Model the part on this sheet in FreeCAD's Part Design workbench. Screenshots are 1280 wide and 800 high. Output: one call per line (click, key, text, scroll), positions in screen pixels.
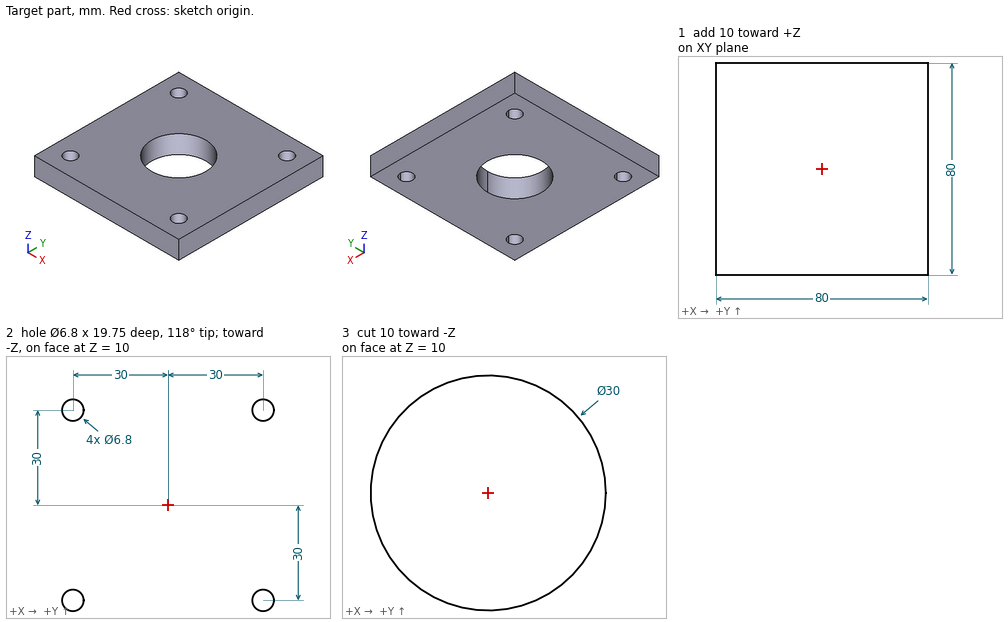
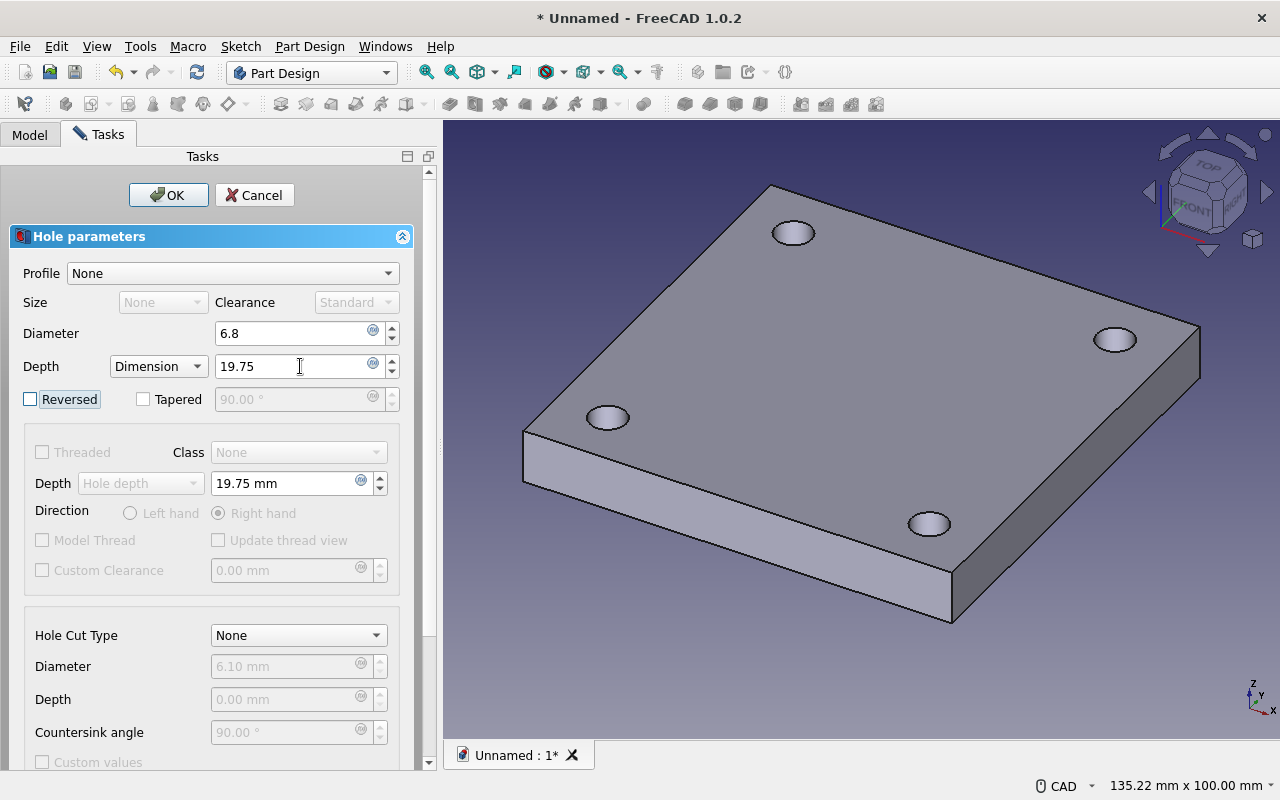
click(169, 195)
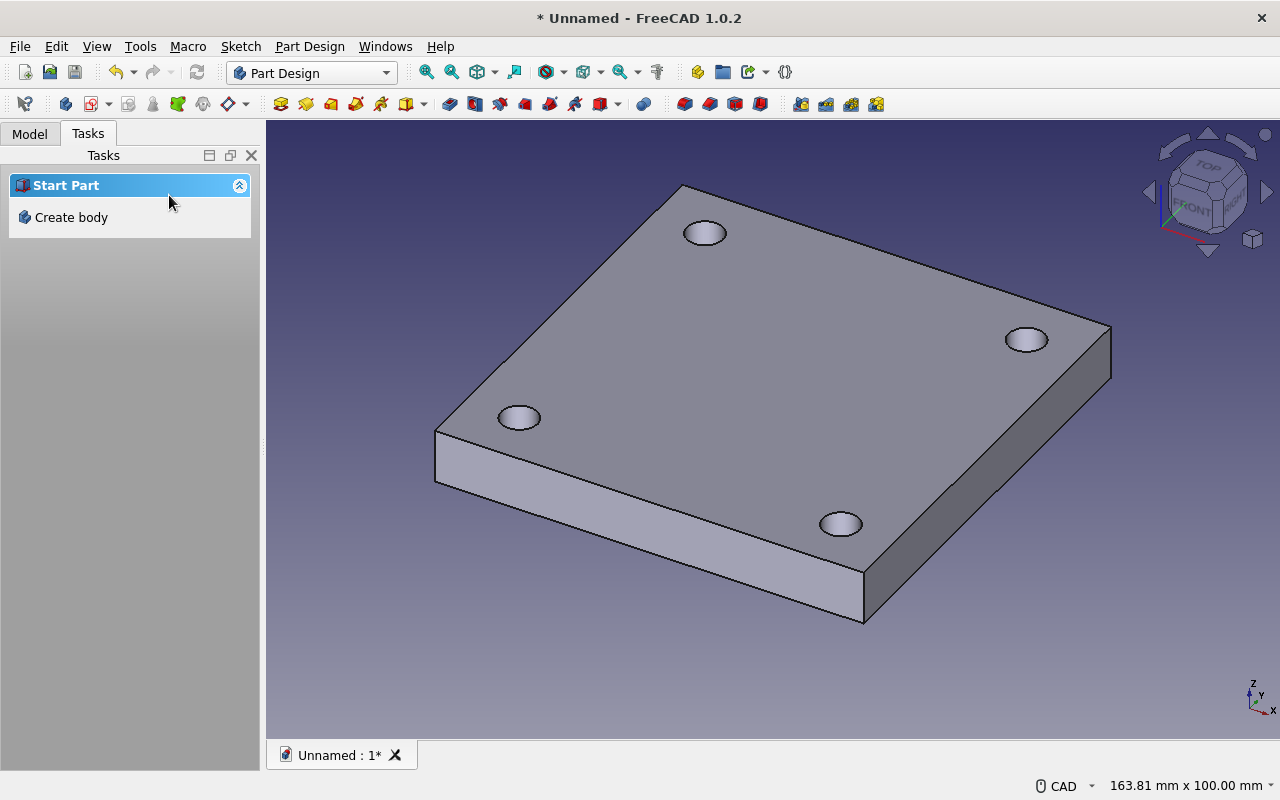
click(773, 378)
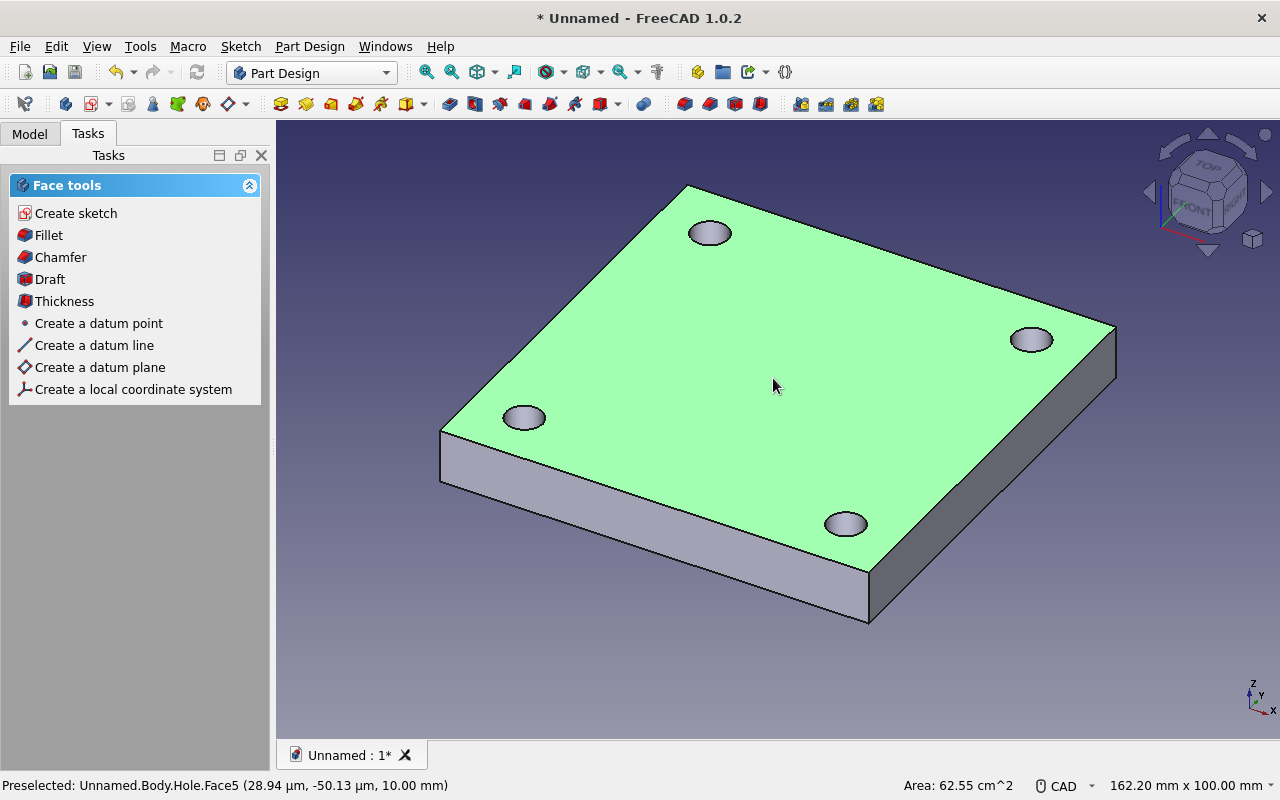
click(90, 104)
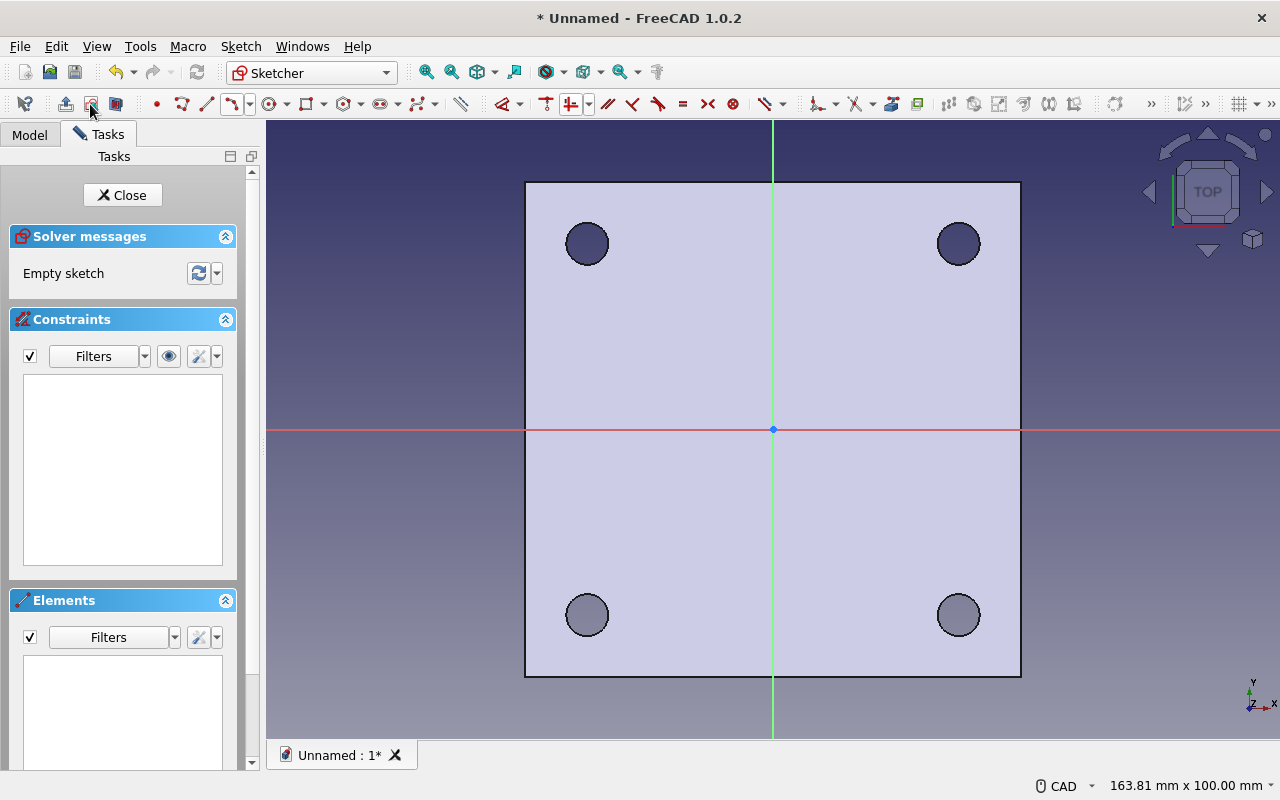
scroll(829, 430, up, 4)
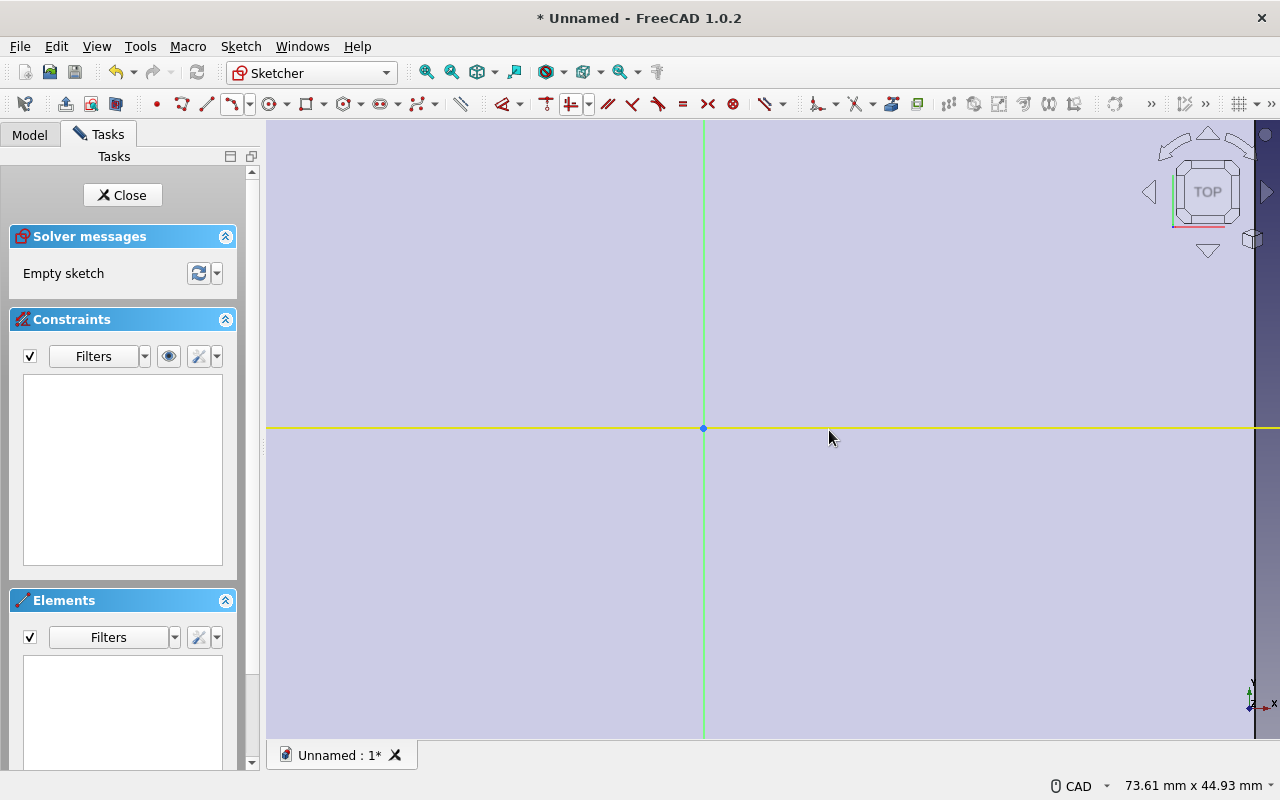
click(268, 104)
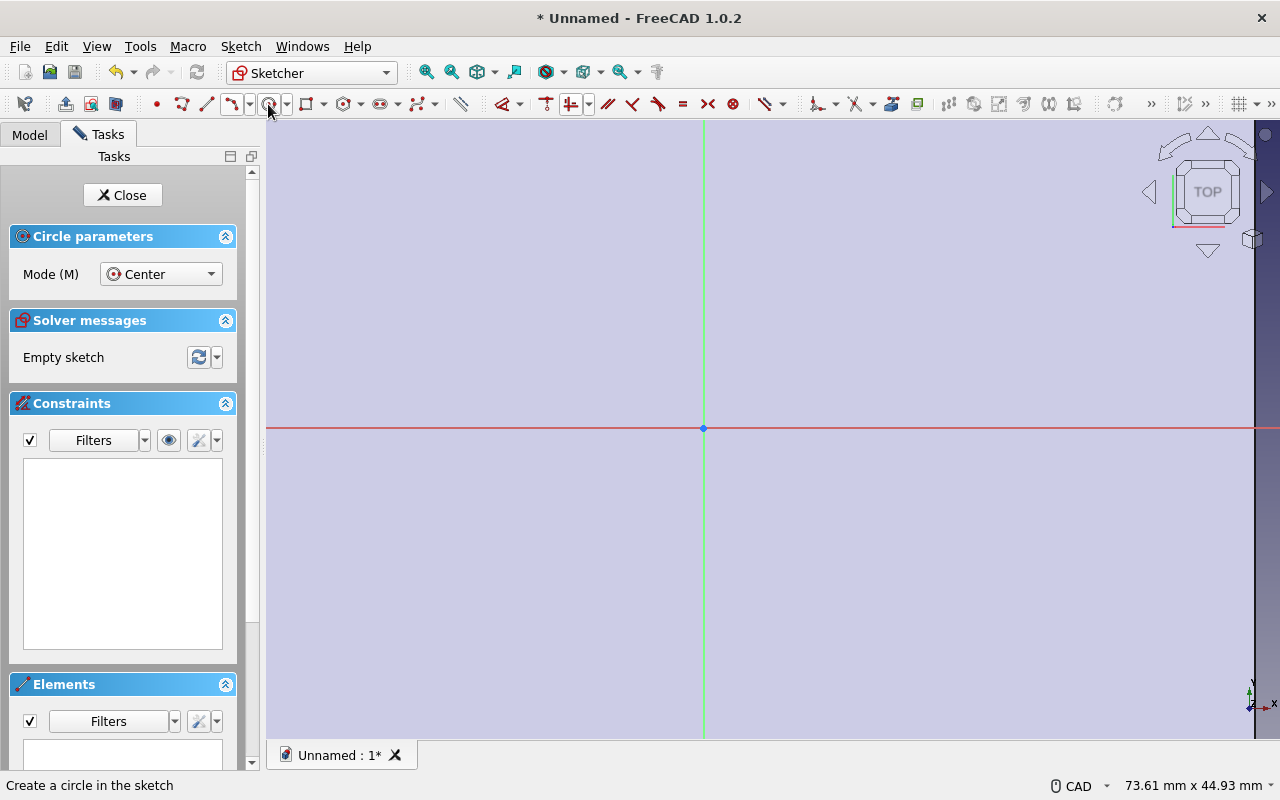
click(704, 428)
move(850, 282)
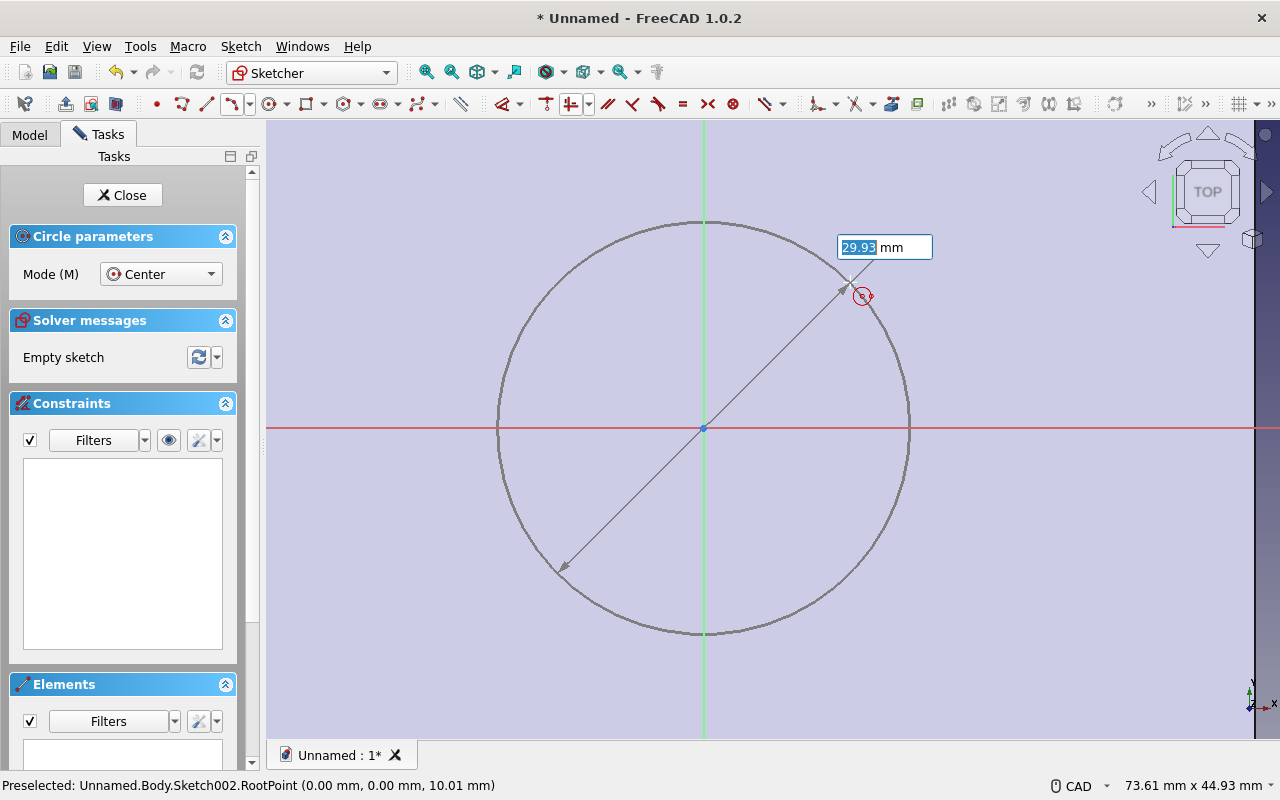
text(30)
key(Return)
key(Escape)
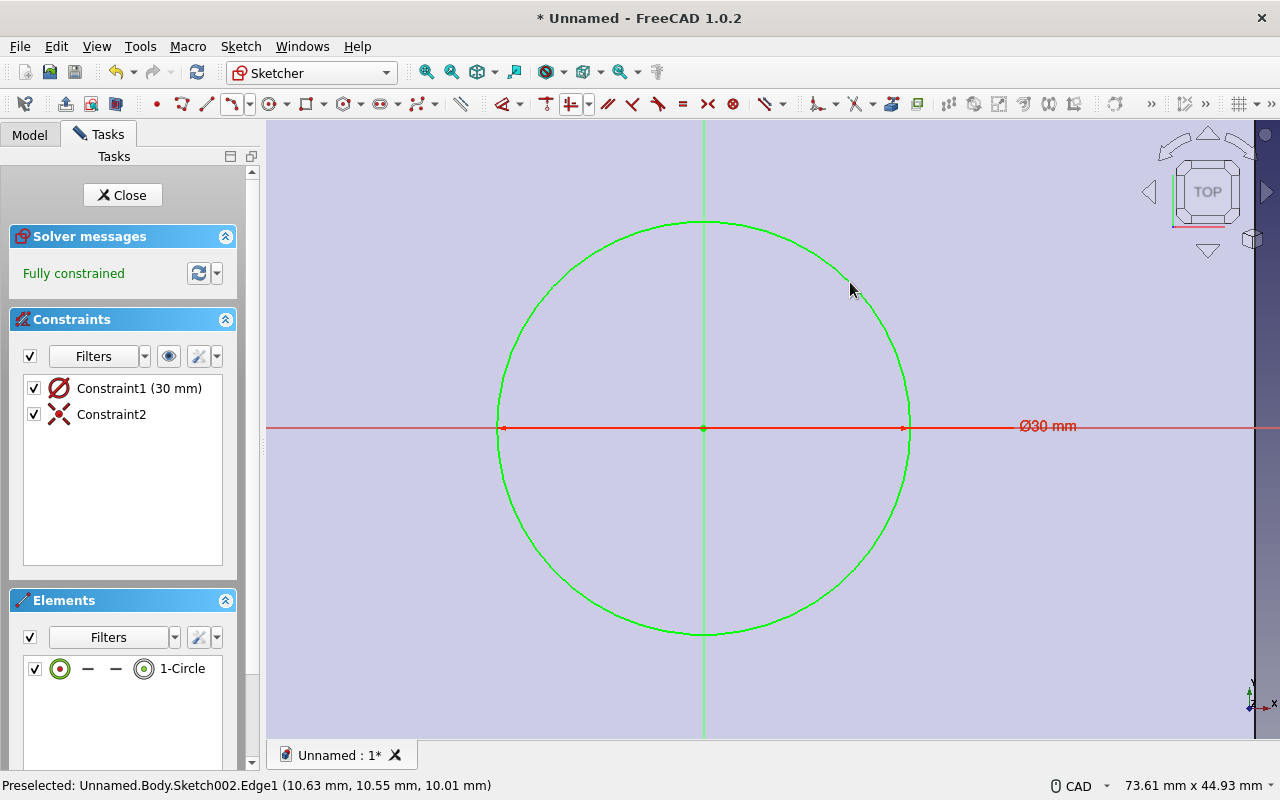
click(123, 195)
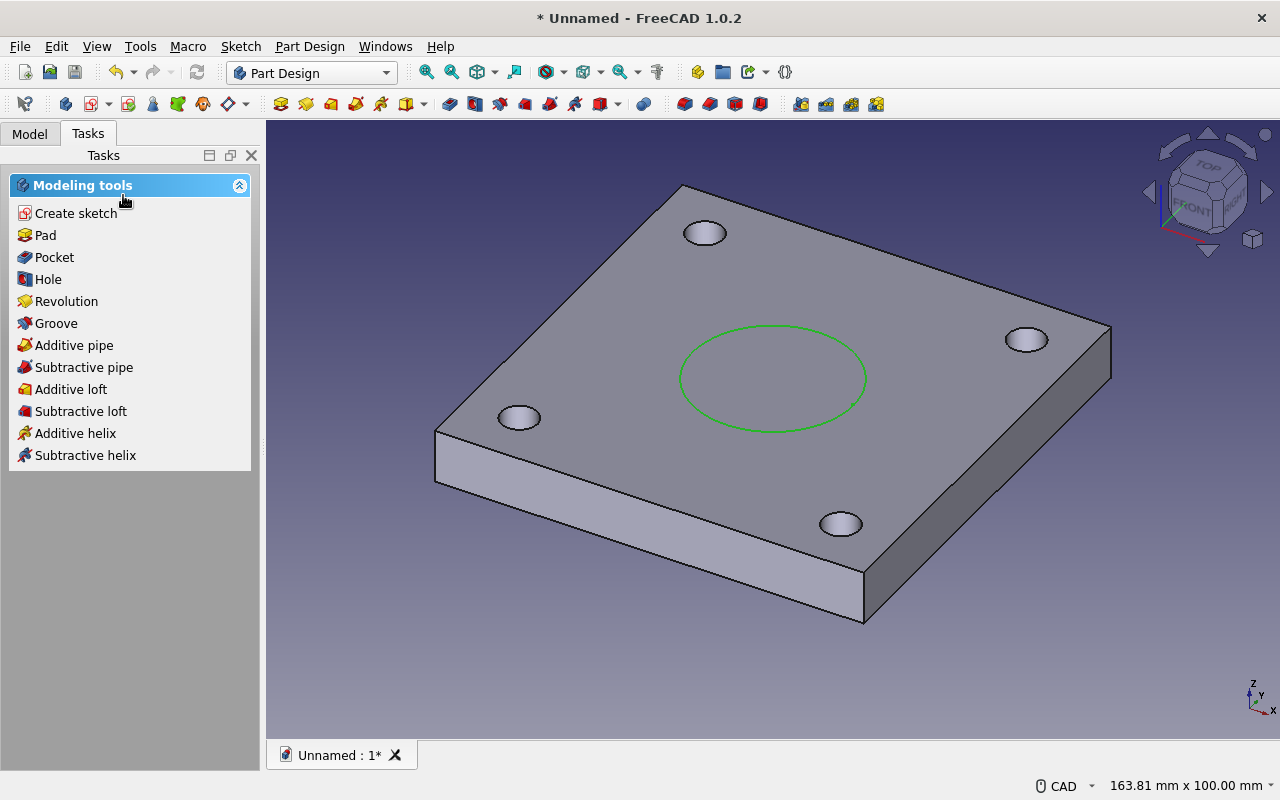
click(450, 104)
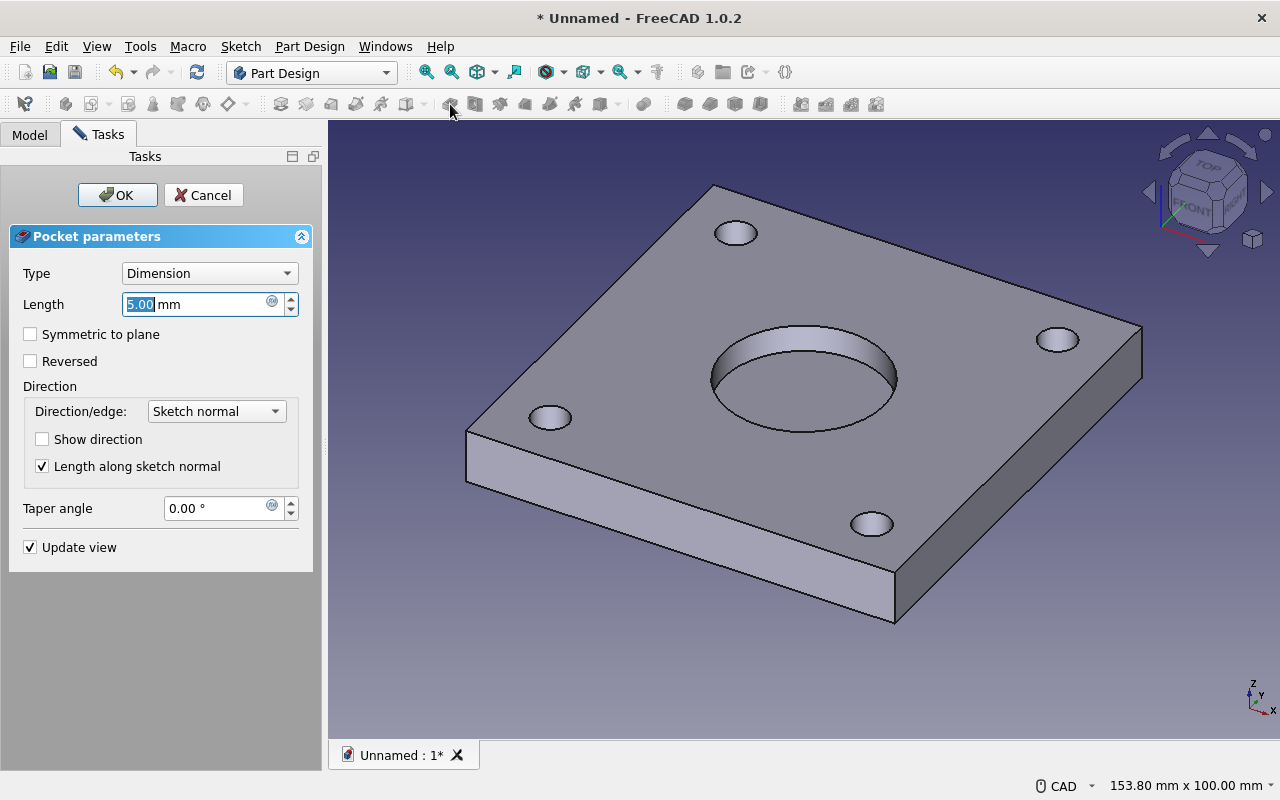
text(10)
key(Tab)